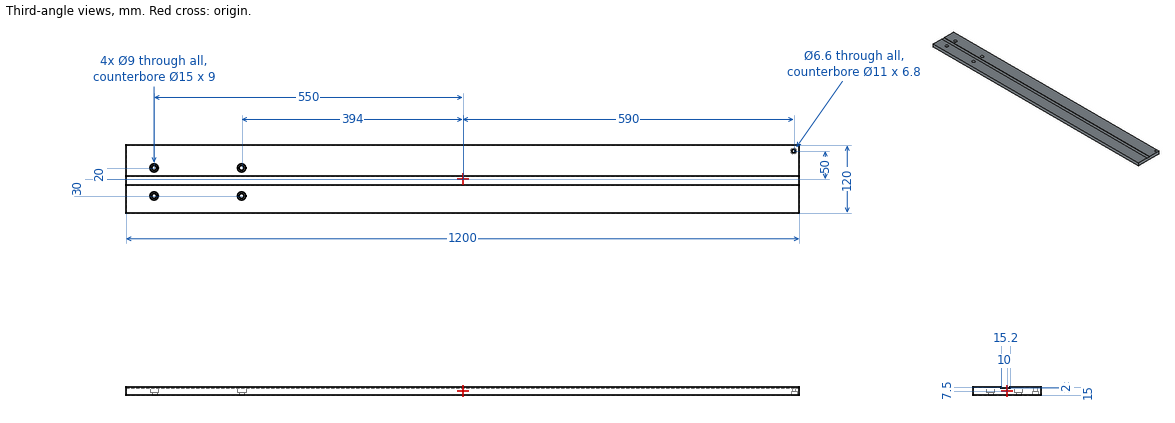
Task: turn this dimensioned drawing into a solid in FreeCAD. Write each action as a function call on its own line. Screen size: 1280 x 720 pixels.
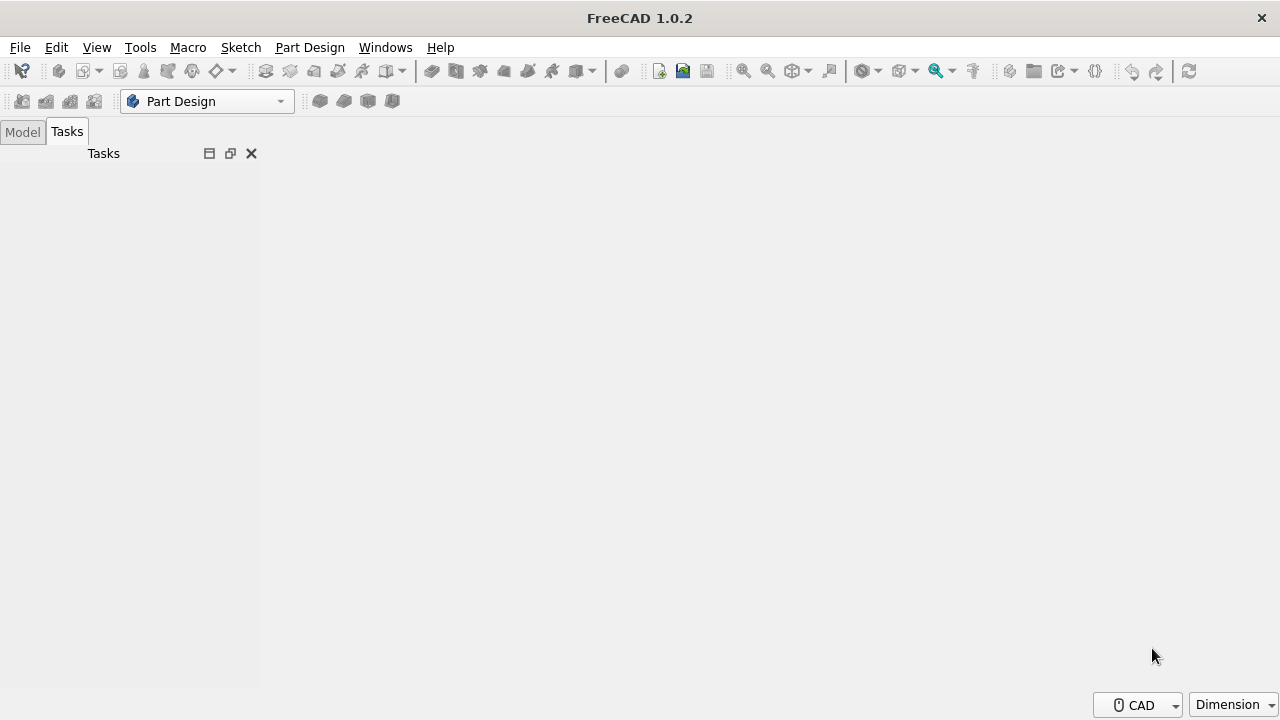
click(660, 72)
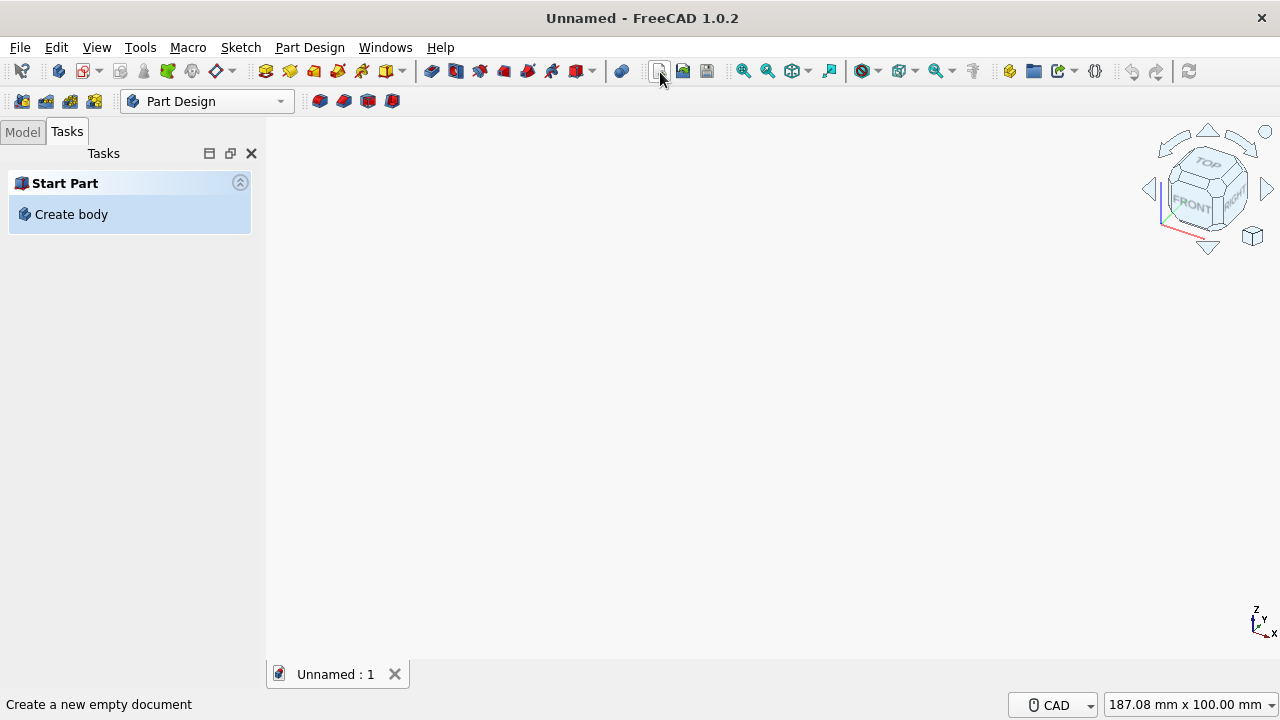
click(84, 72)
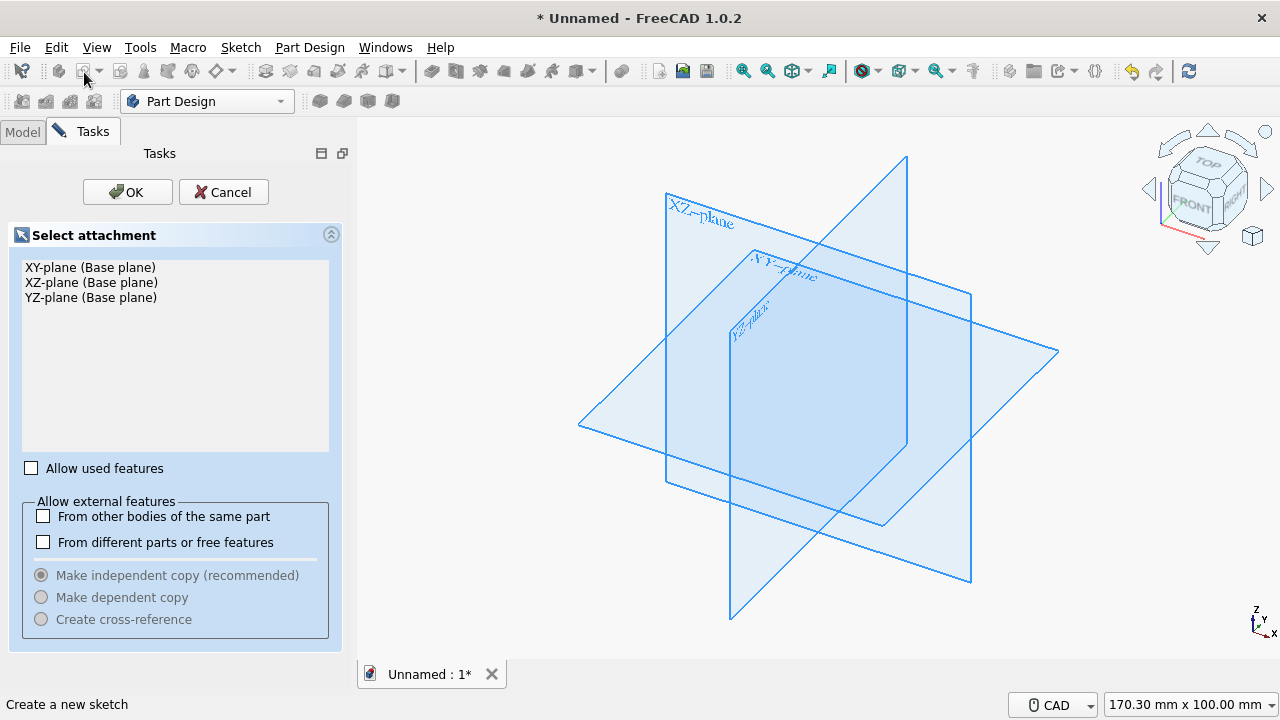
click(82, 268)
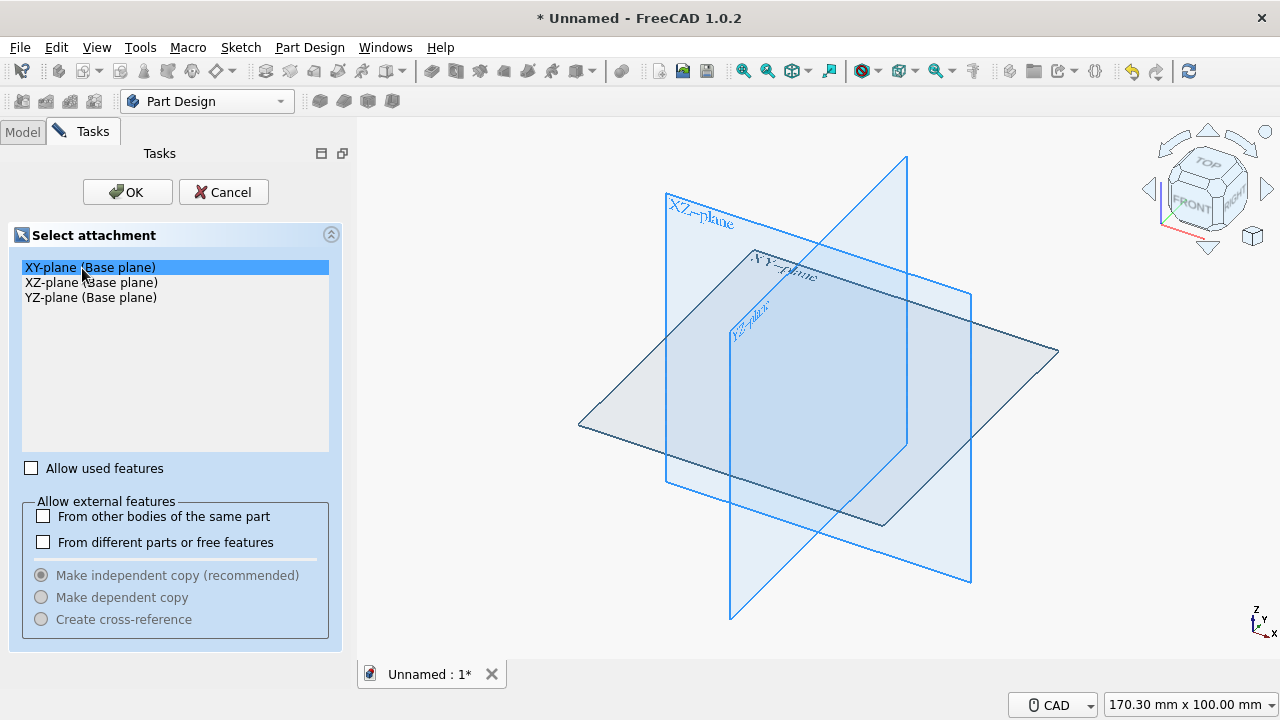
click(128, 192)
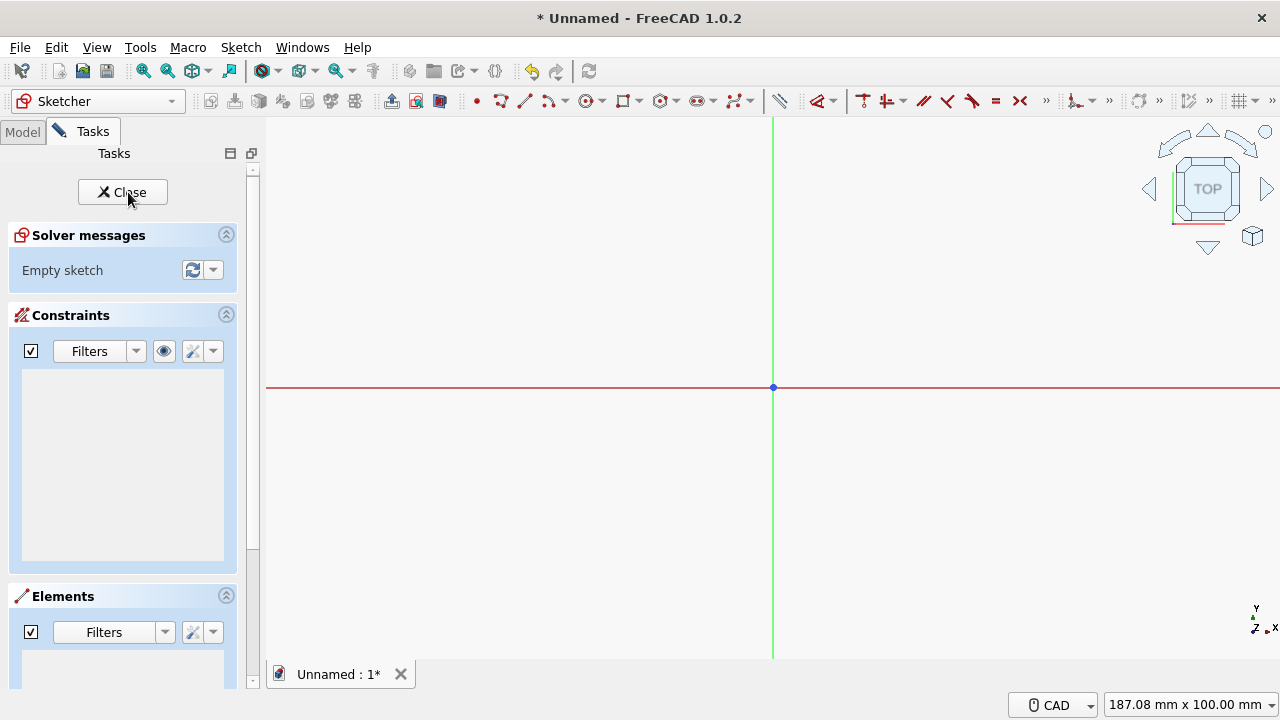
scroll(698, 388, down, 12)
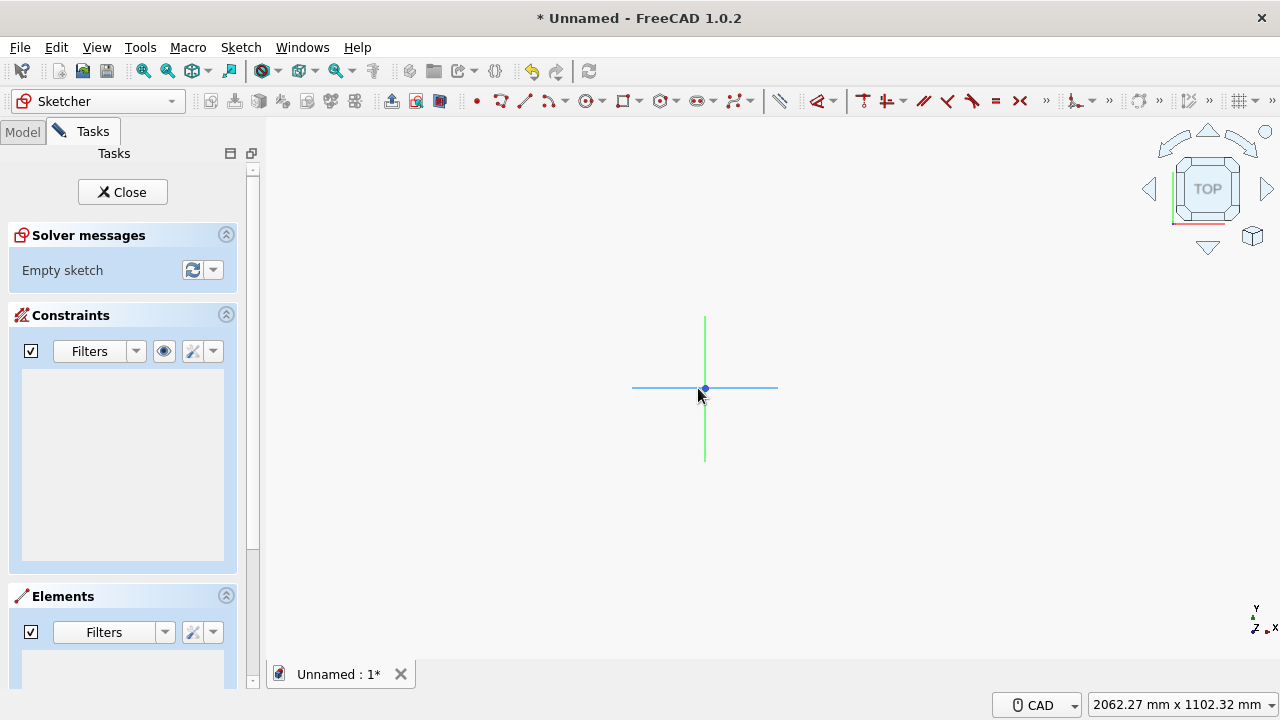
key(g)
key(v)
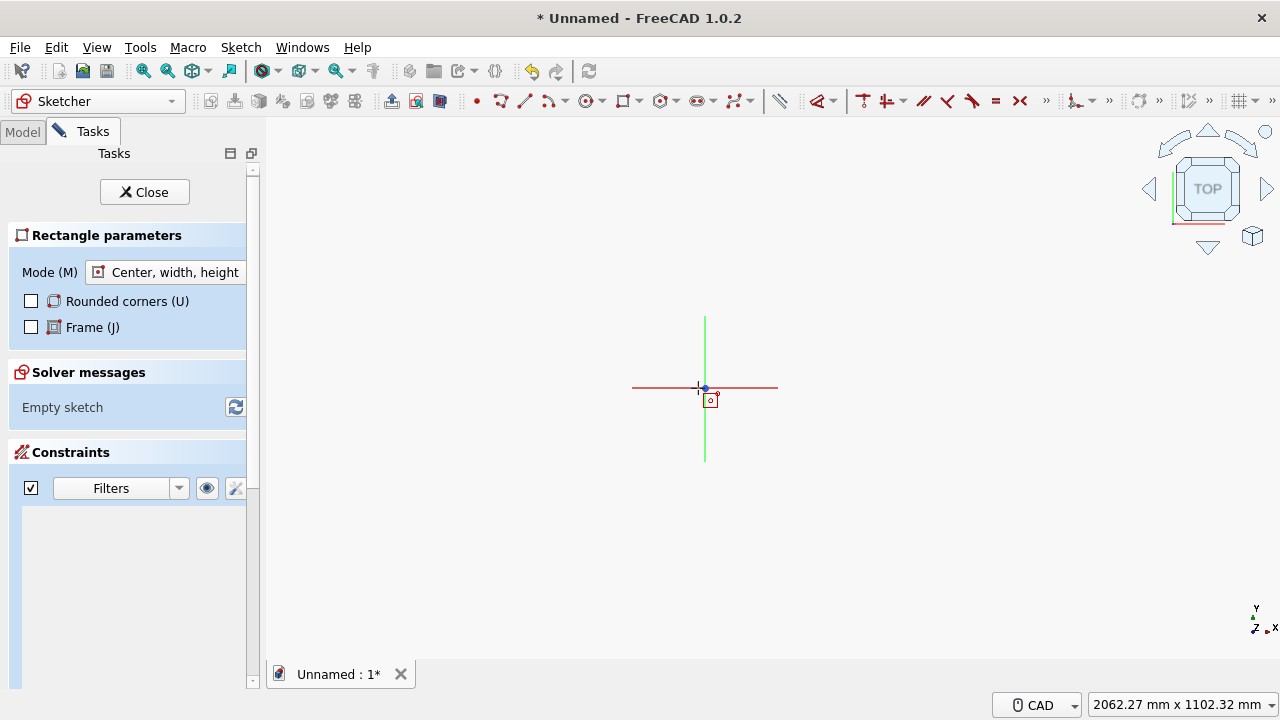
click(705, 388)
move(1000, 359)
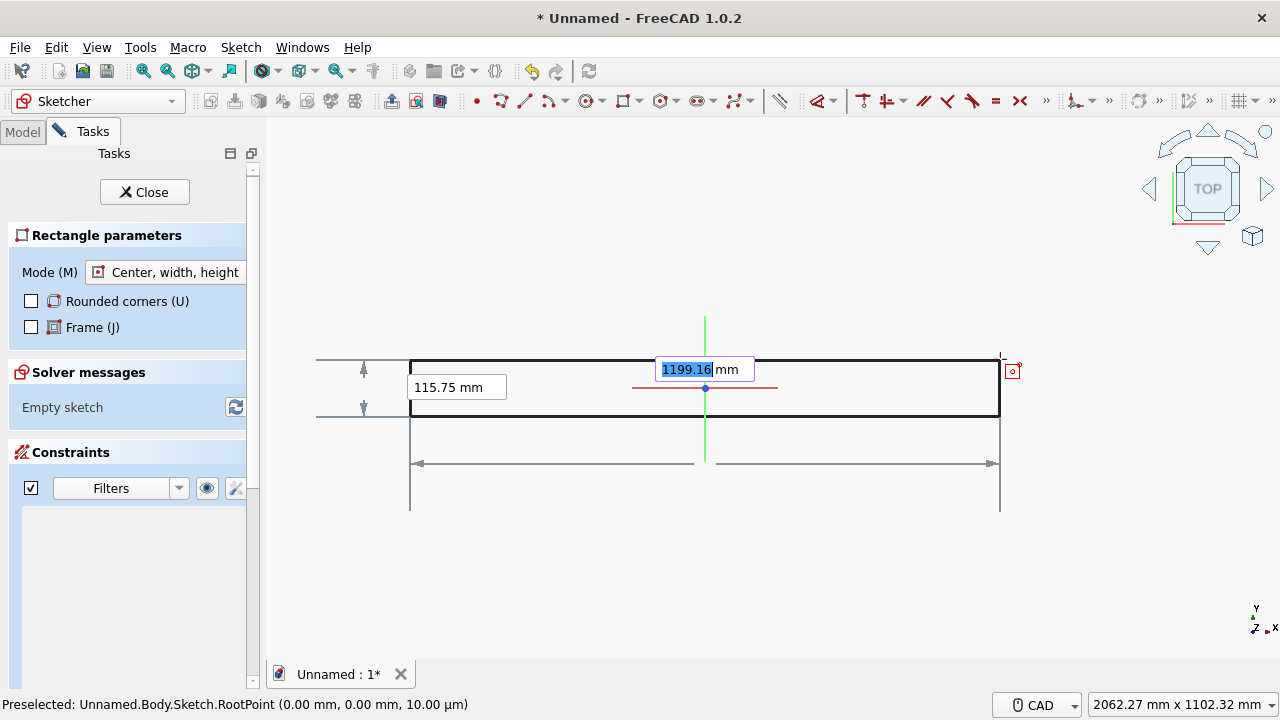
text(1200)
key(Tab)
text(120)
key(Return)
key(Escape)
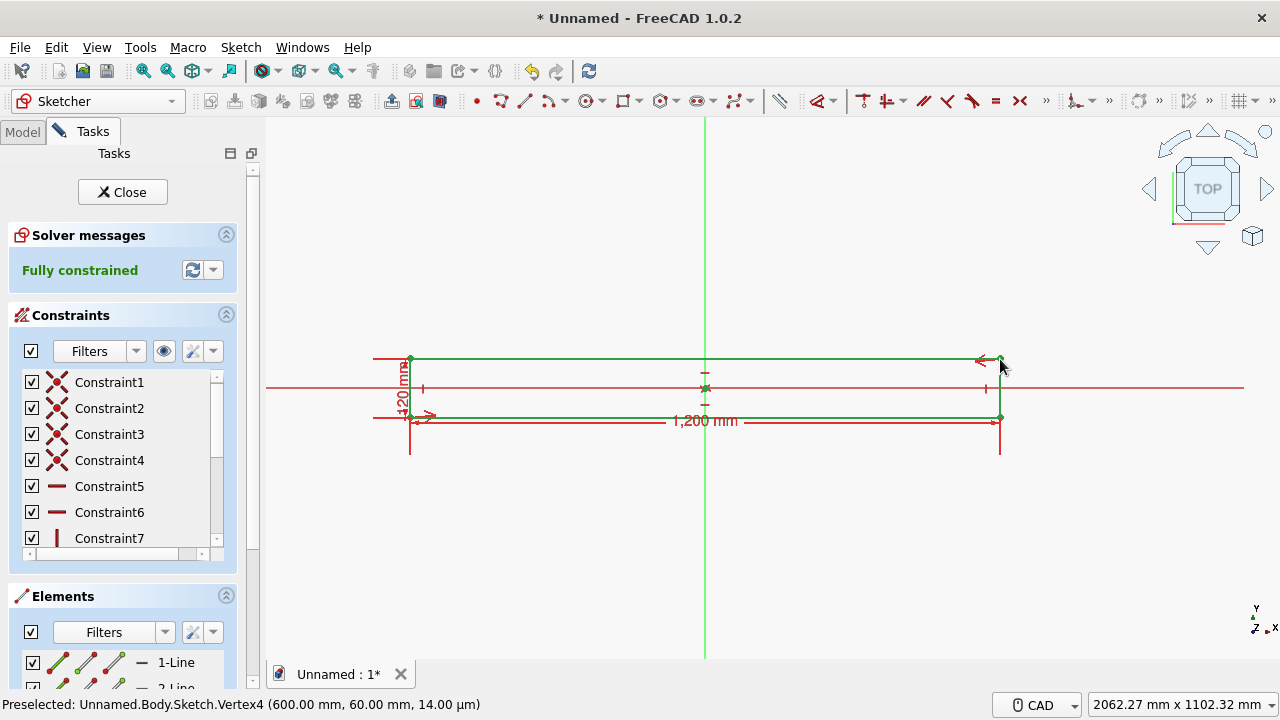
click(123, 192)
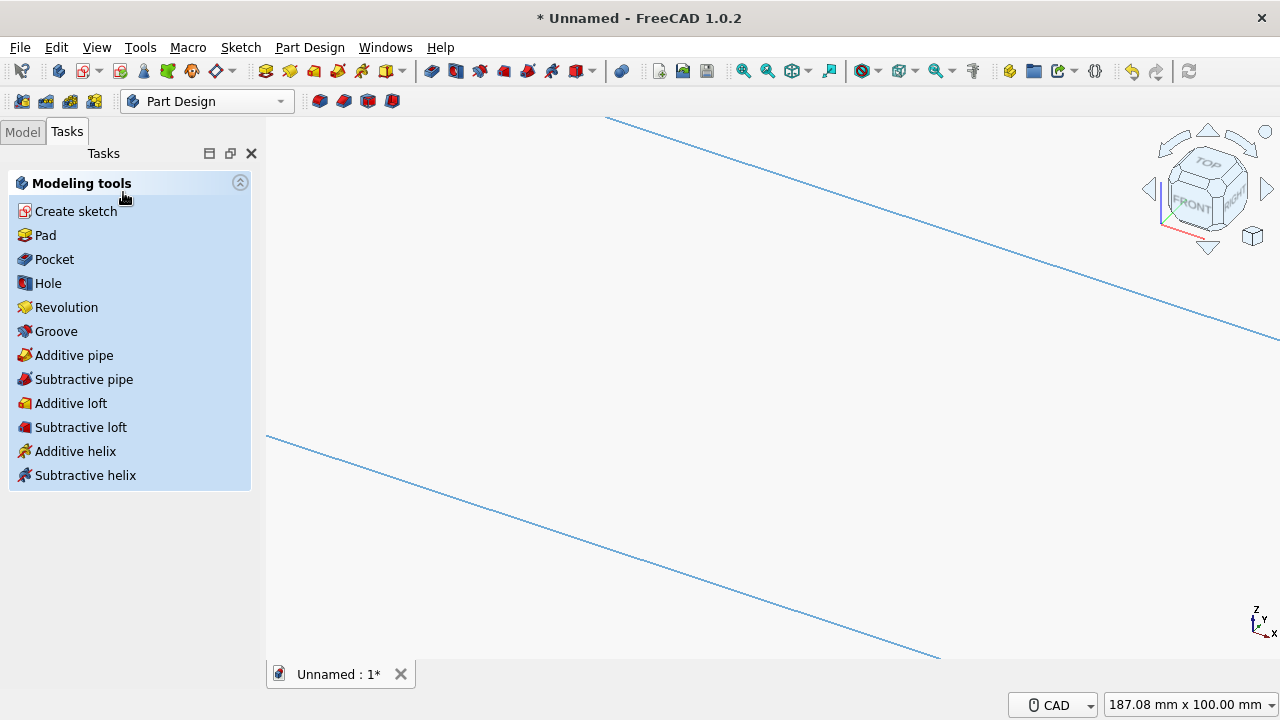
click(266, 72)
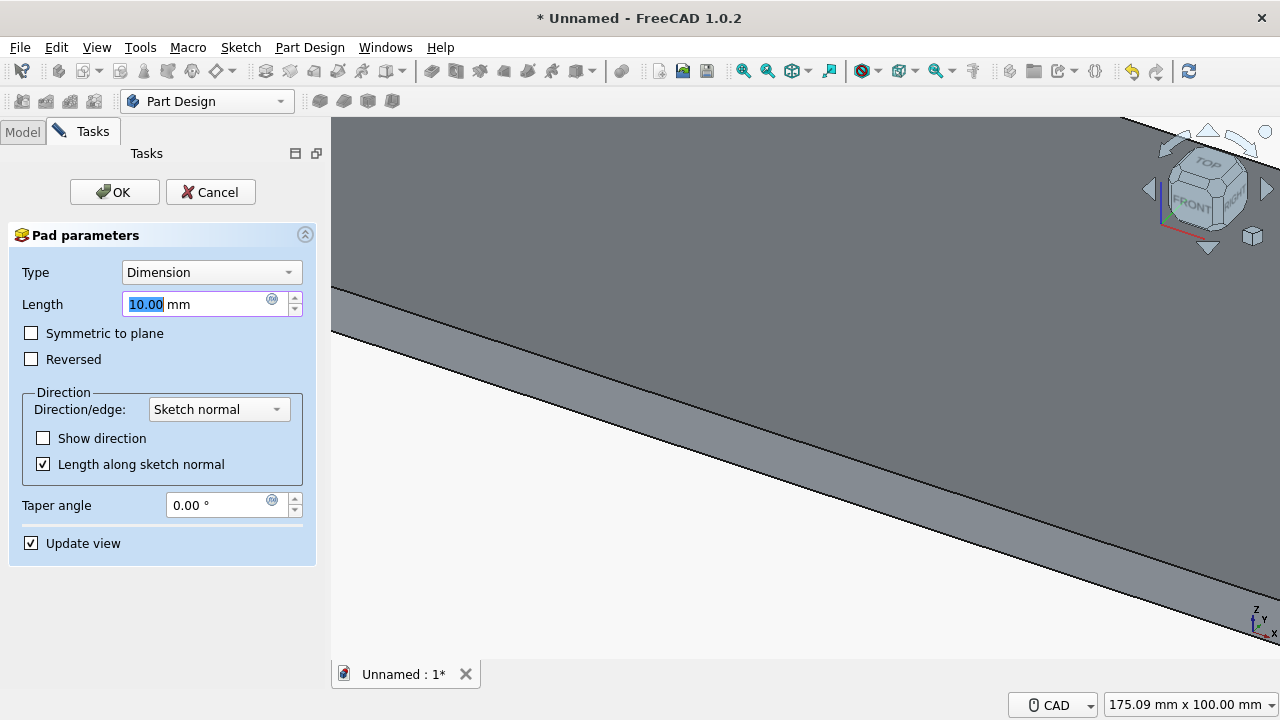
text(15)
key(Tab)